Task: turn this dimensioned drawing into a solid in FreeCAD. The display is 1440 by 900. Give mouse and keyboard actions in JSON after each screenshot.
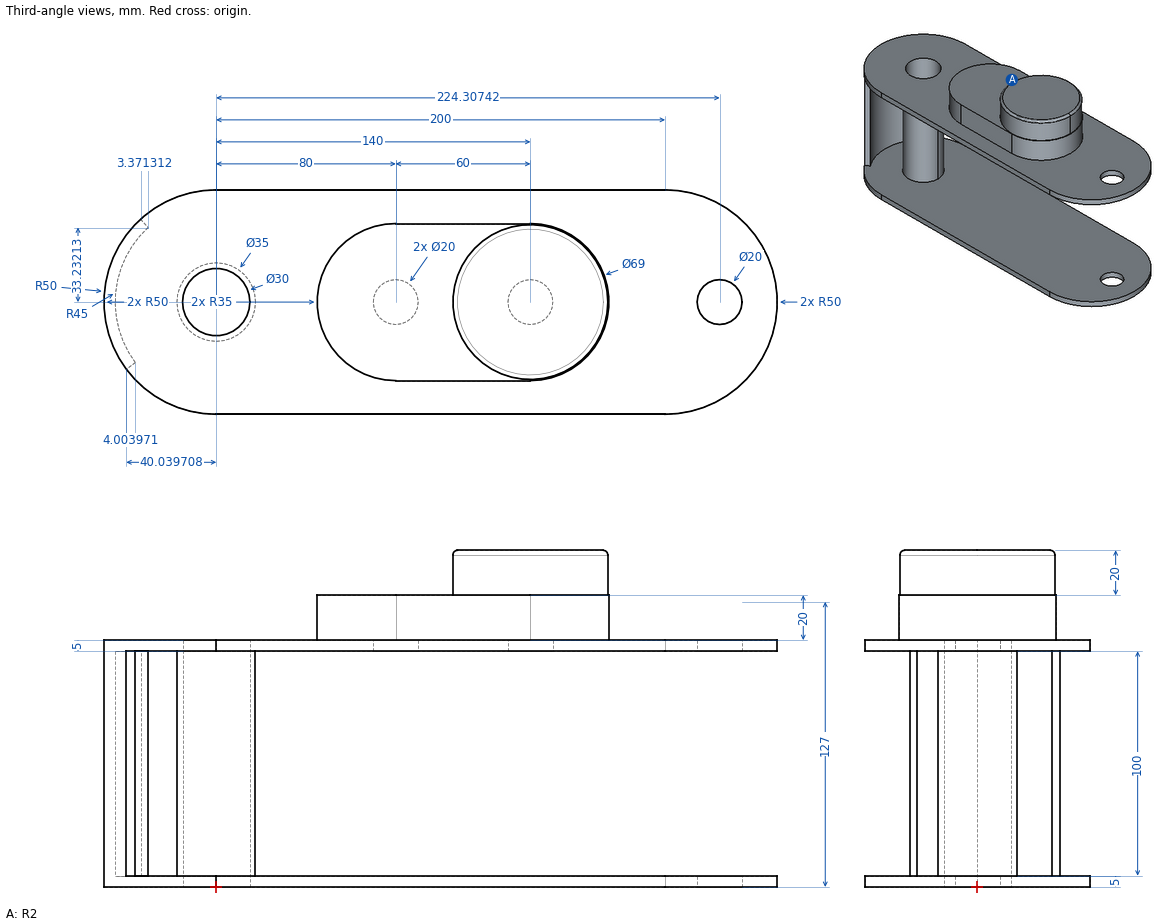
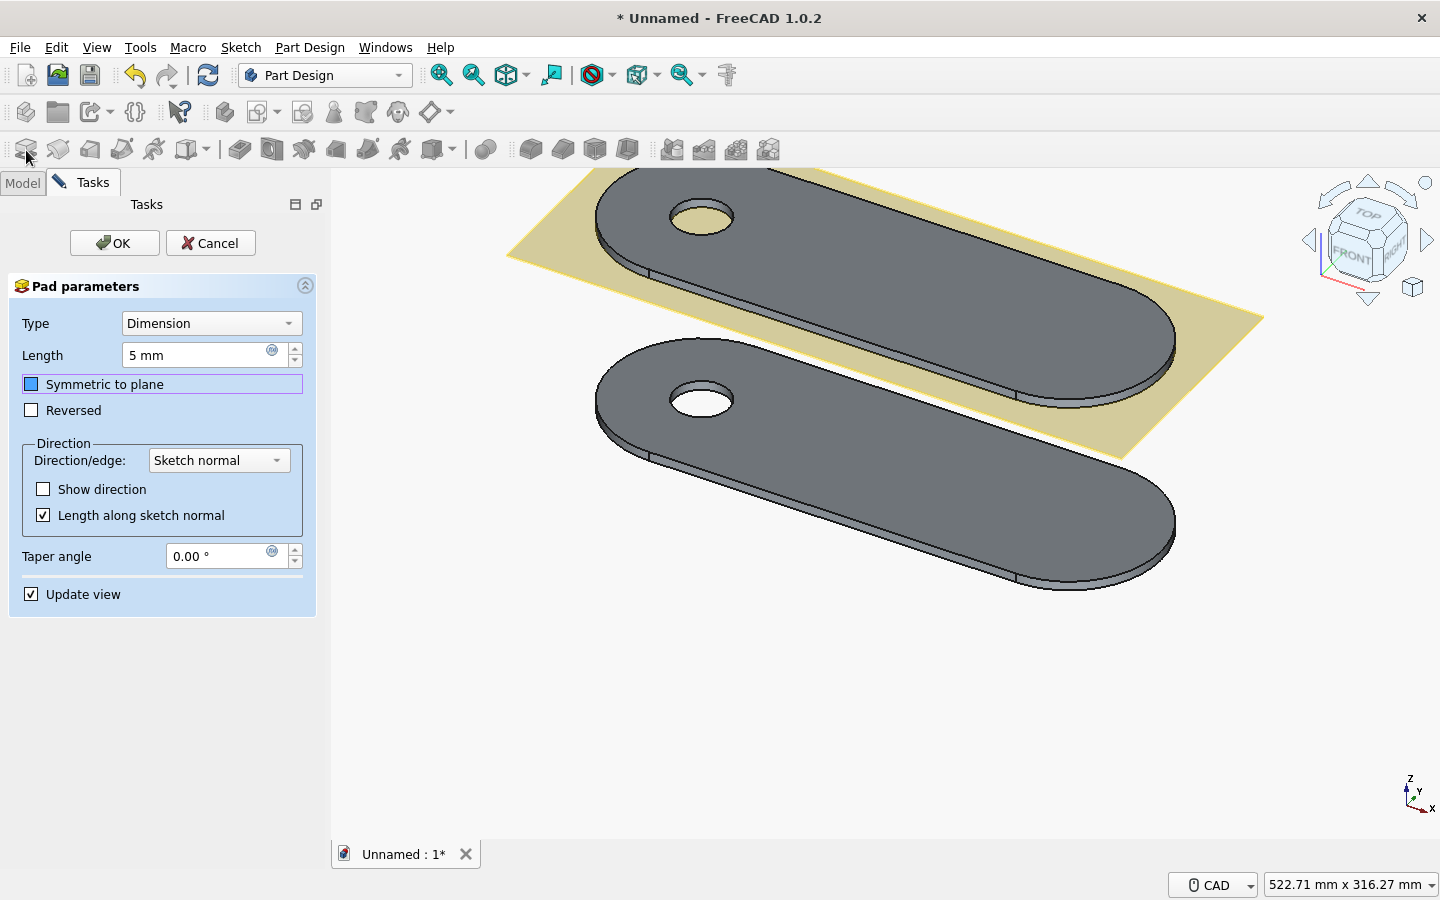
{"action": "left_click", "coordinate": [115, 243]}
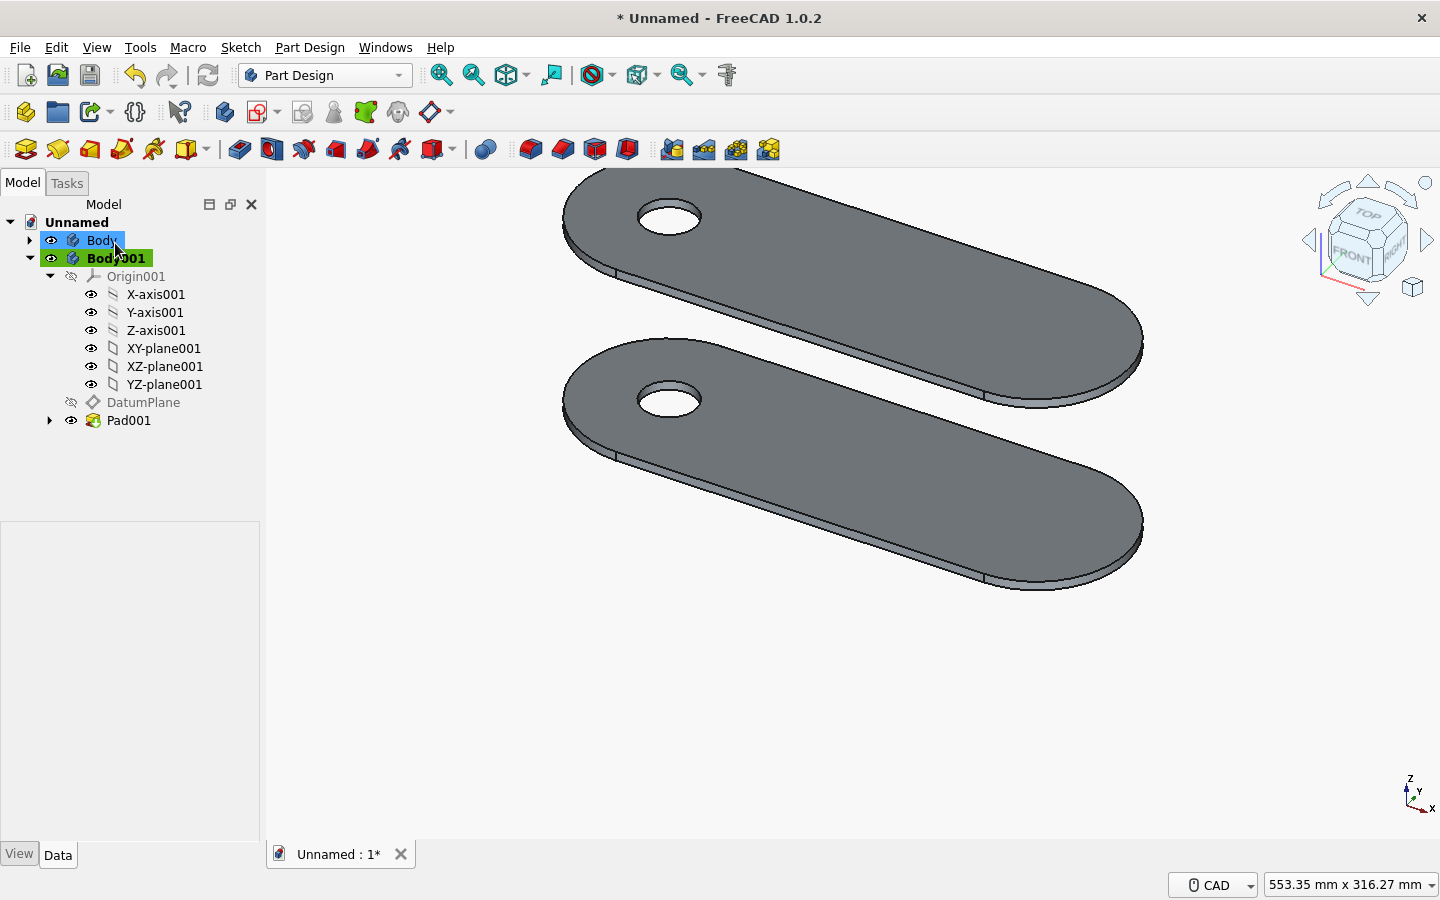
{"action": "left_click", "coordinate": [442, 76]}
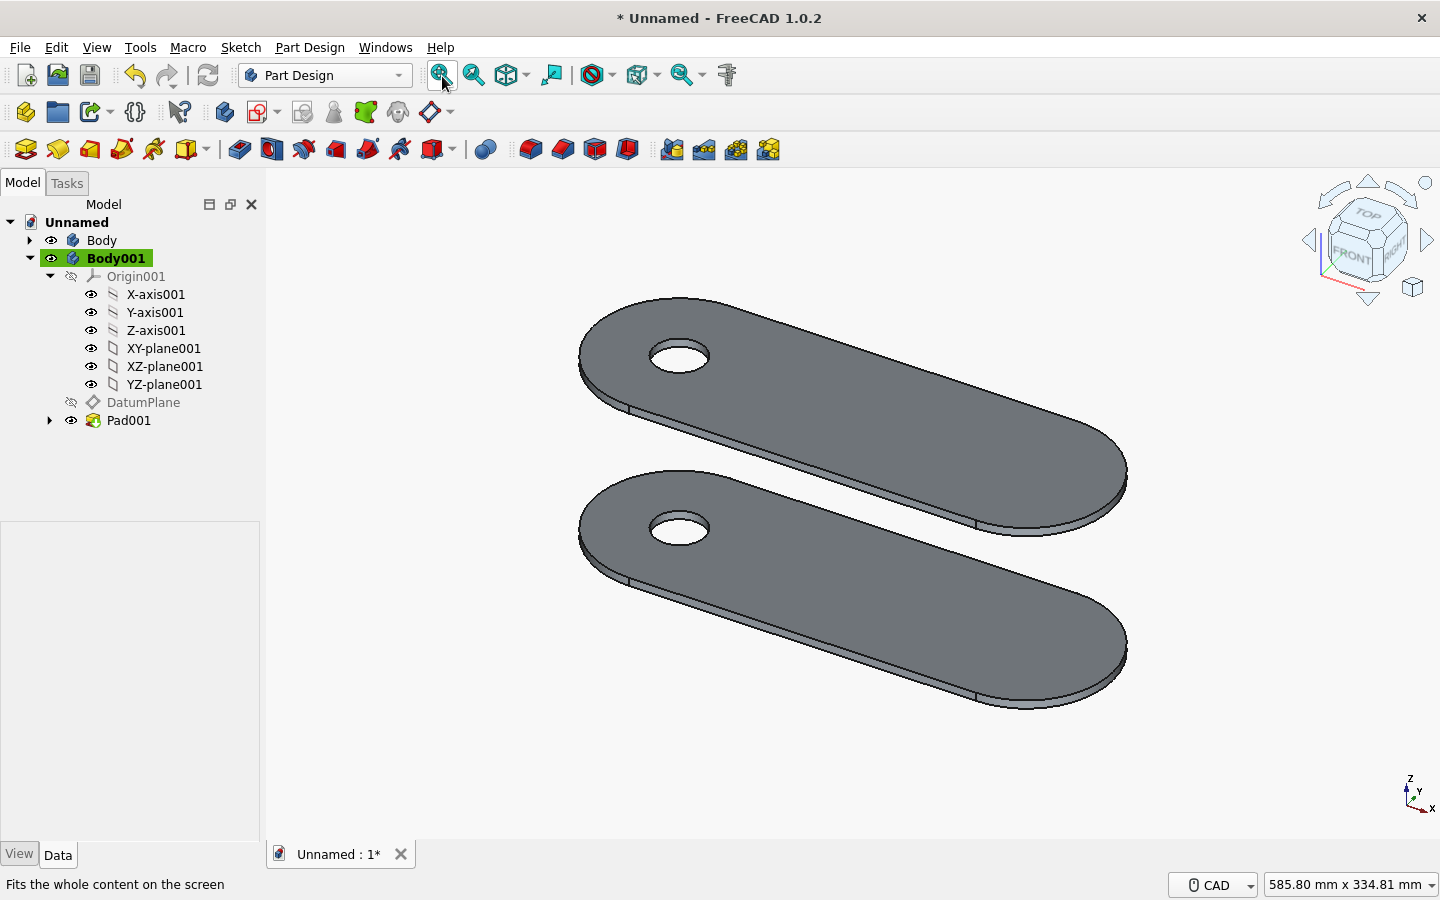
{"action": "double_click", "coordinate": [96, 240]}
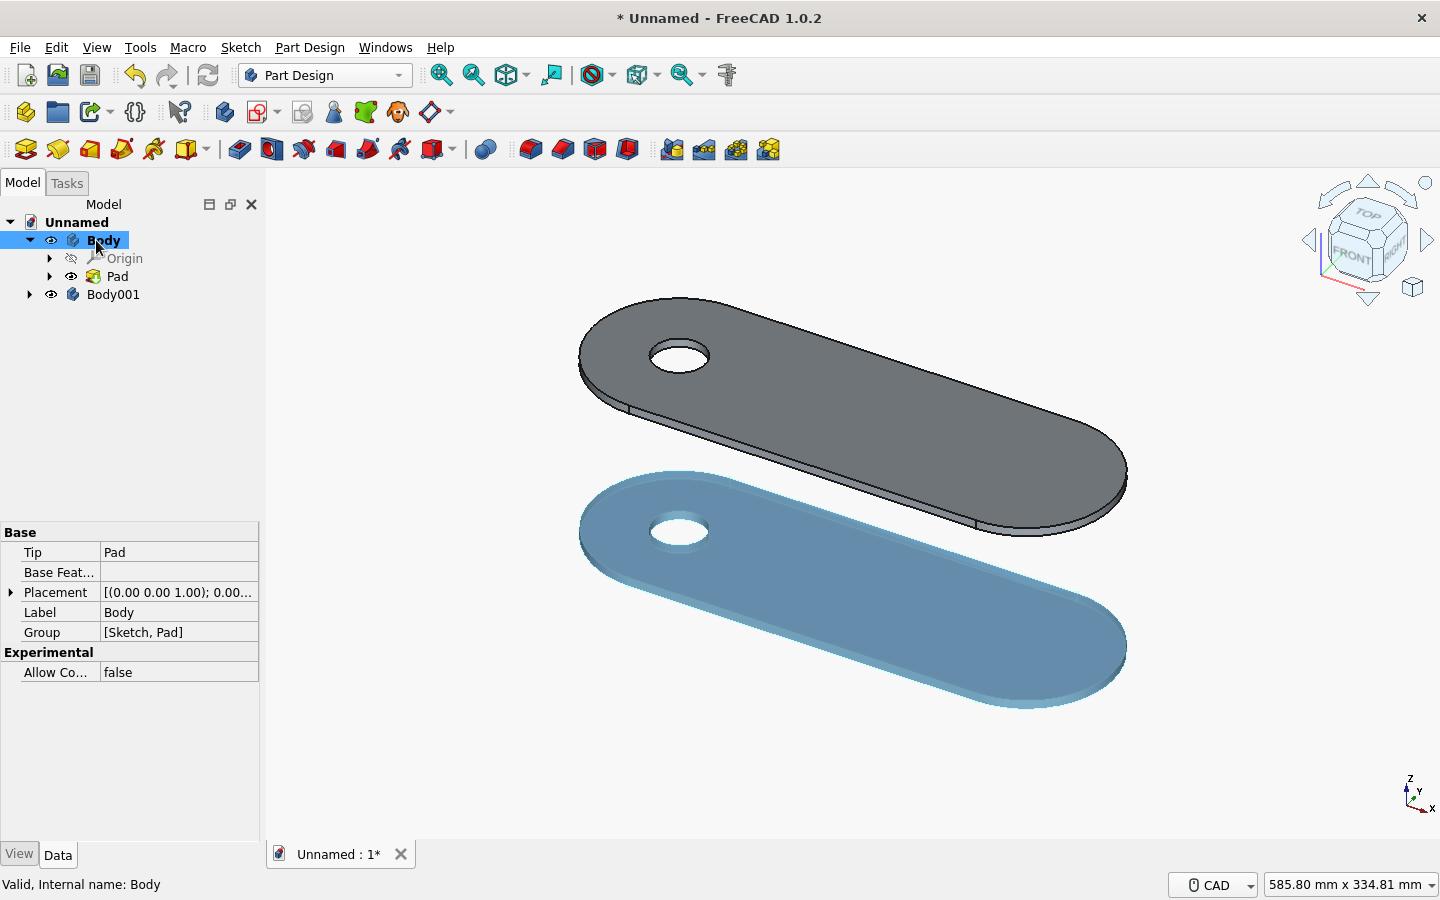
{"action": "left_click", "coordinate": [96, 240]}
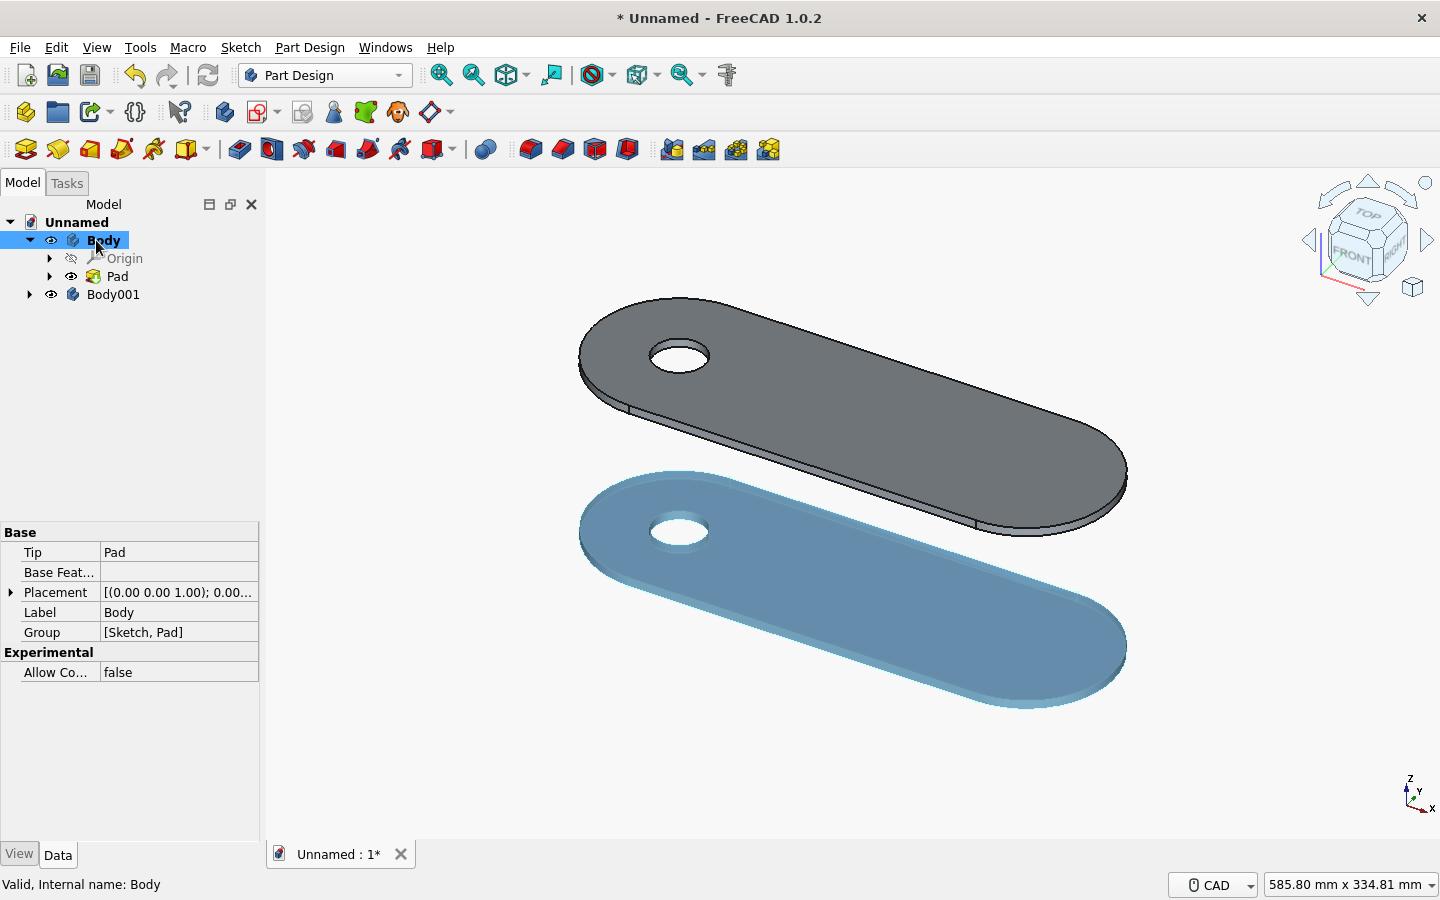
{"action": "left_click", "coordinate": [146, 672]}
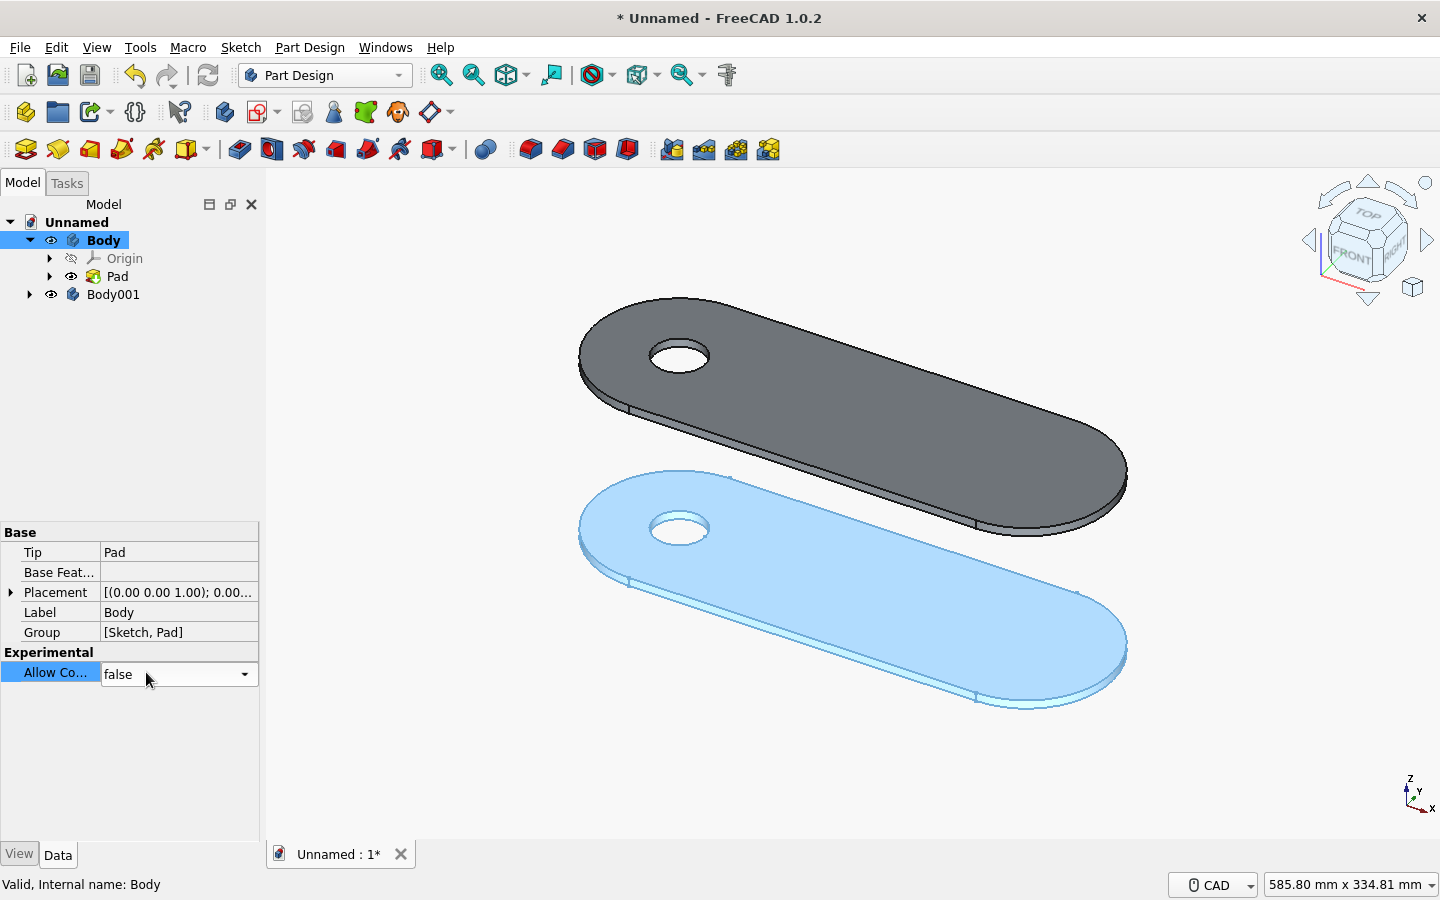
{"action": "left_click", "coordinate": [146, 672]}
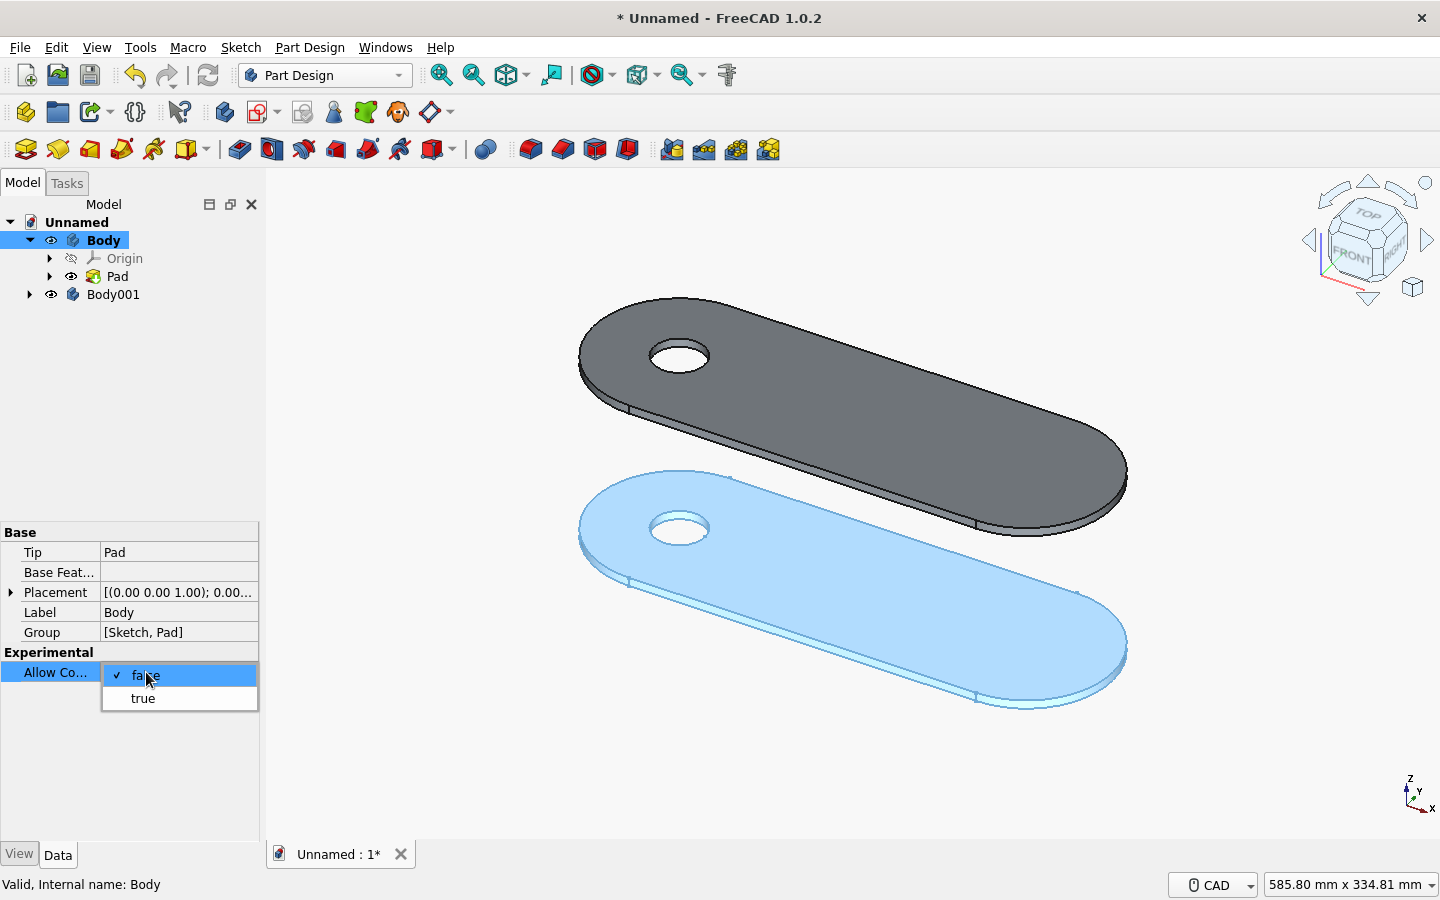
{"action": "left_click", "coordinate": [179, 698]}
{"action": "key", "text": "Return"}